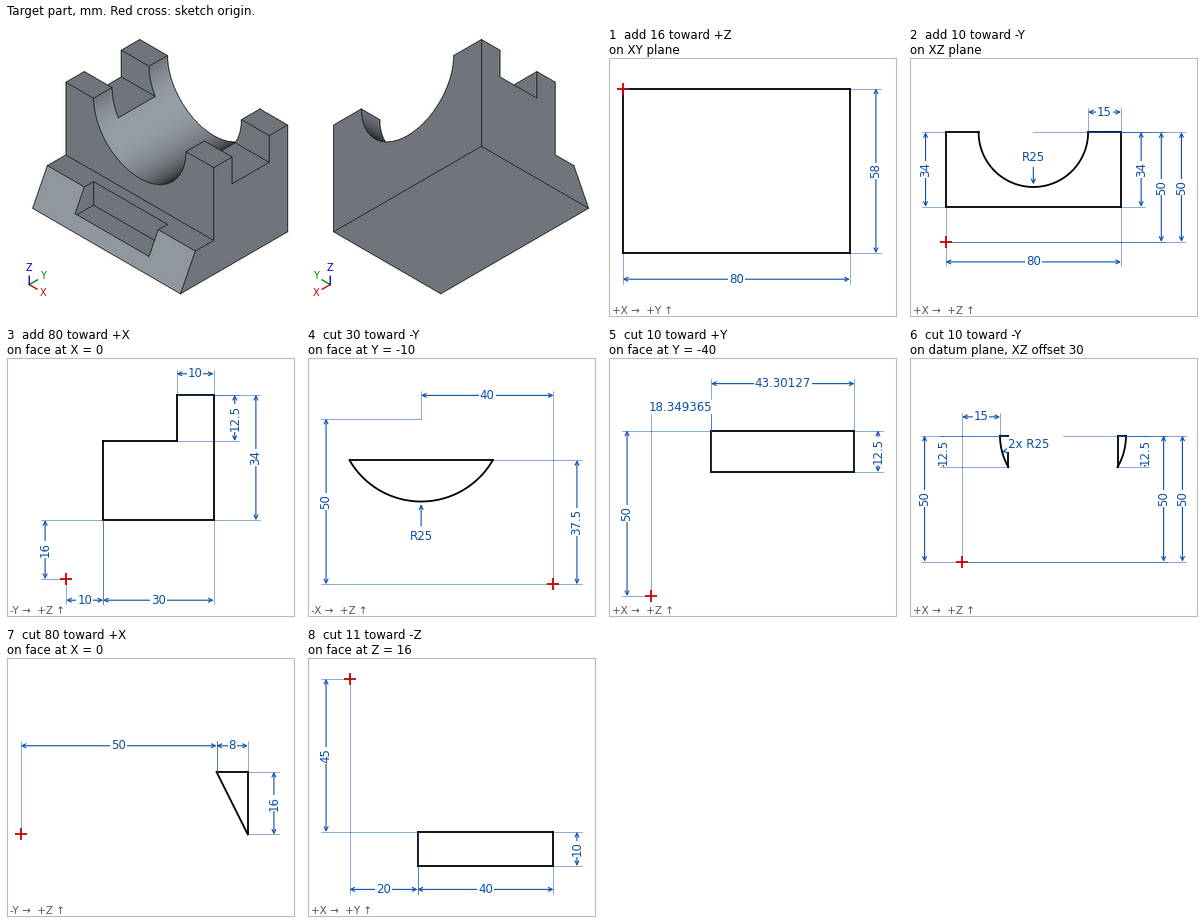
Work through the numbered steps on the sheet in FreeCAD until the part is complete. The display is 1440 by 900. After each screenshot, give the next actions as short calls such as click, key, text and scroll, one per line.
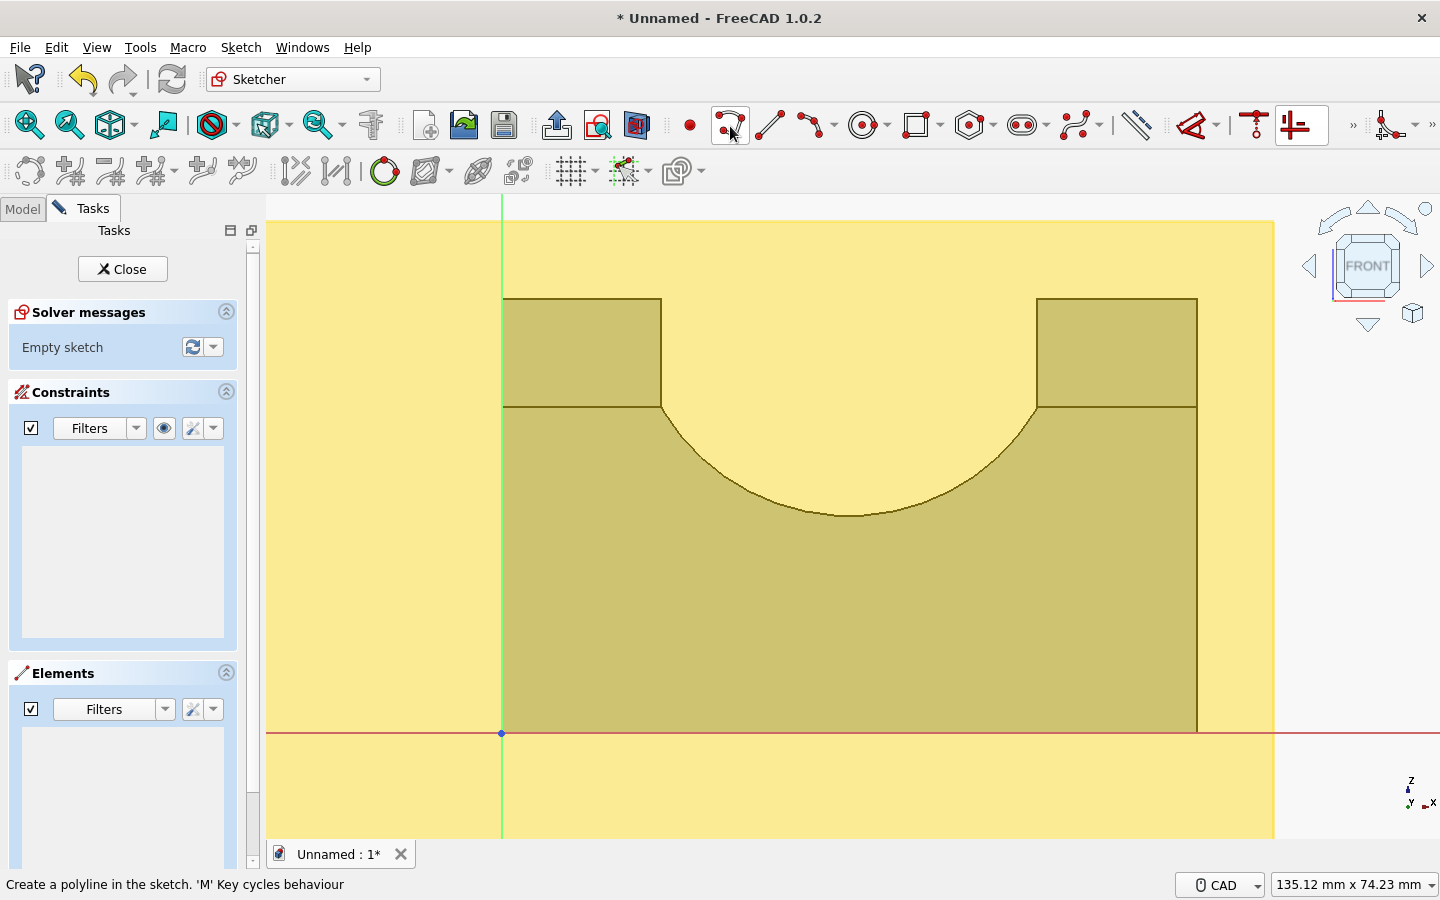
click(632, 299)
click(661, 299)
click(661, 407)
right_click(661, 407)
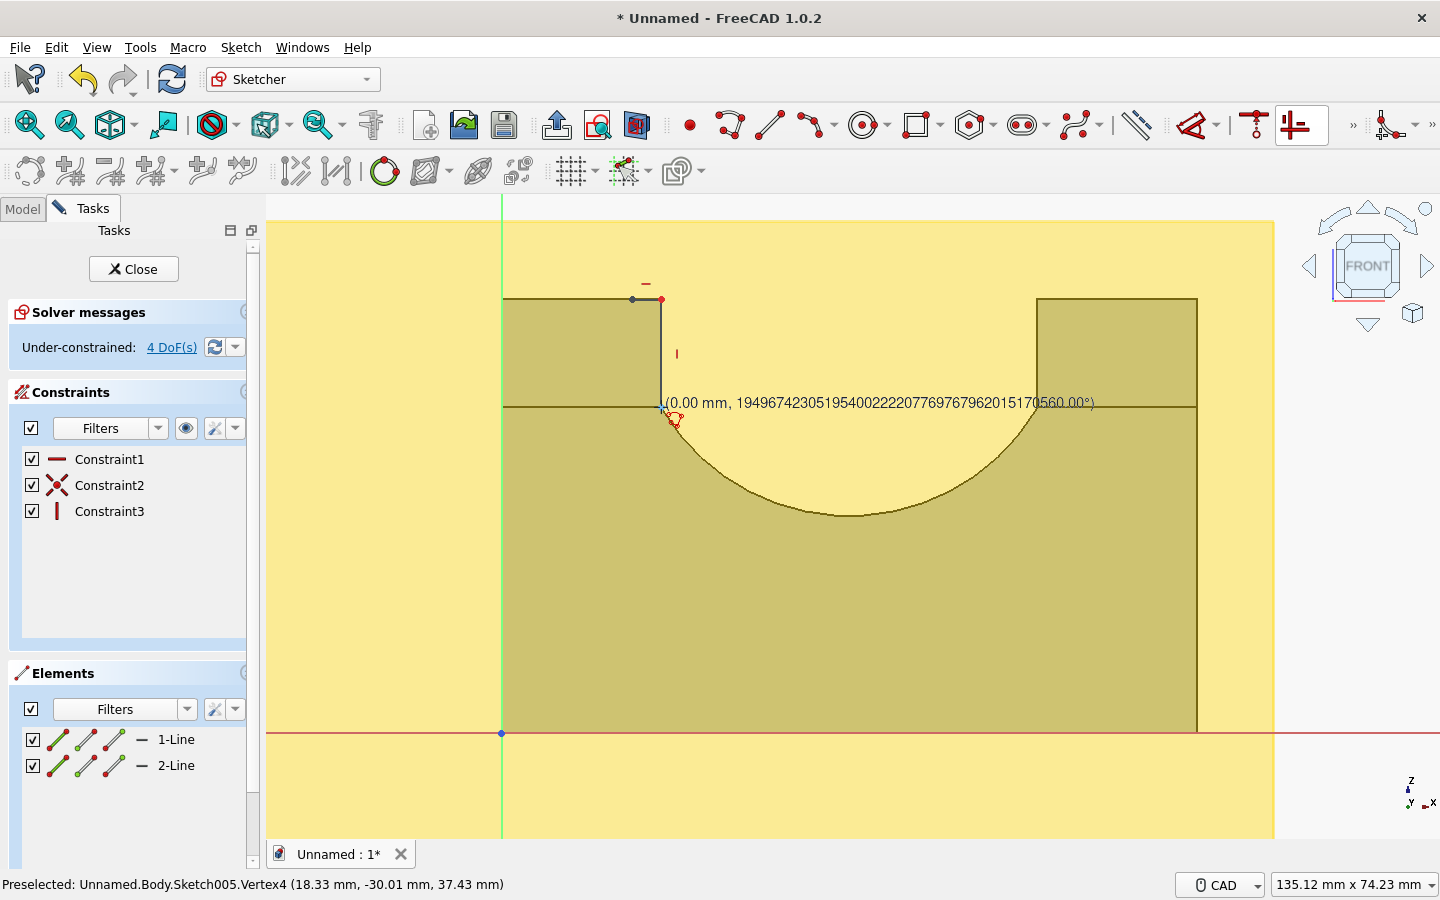
click(810, 126)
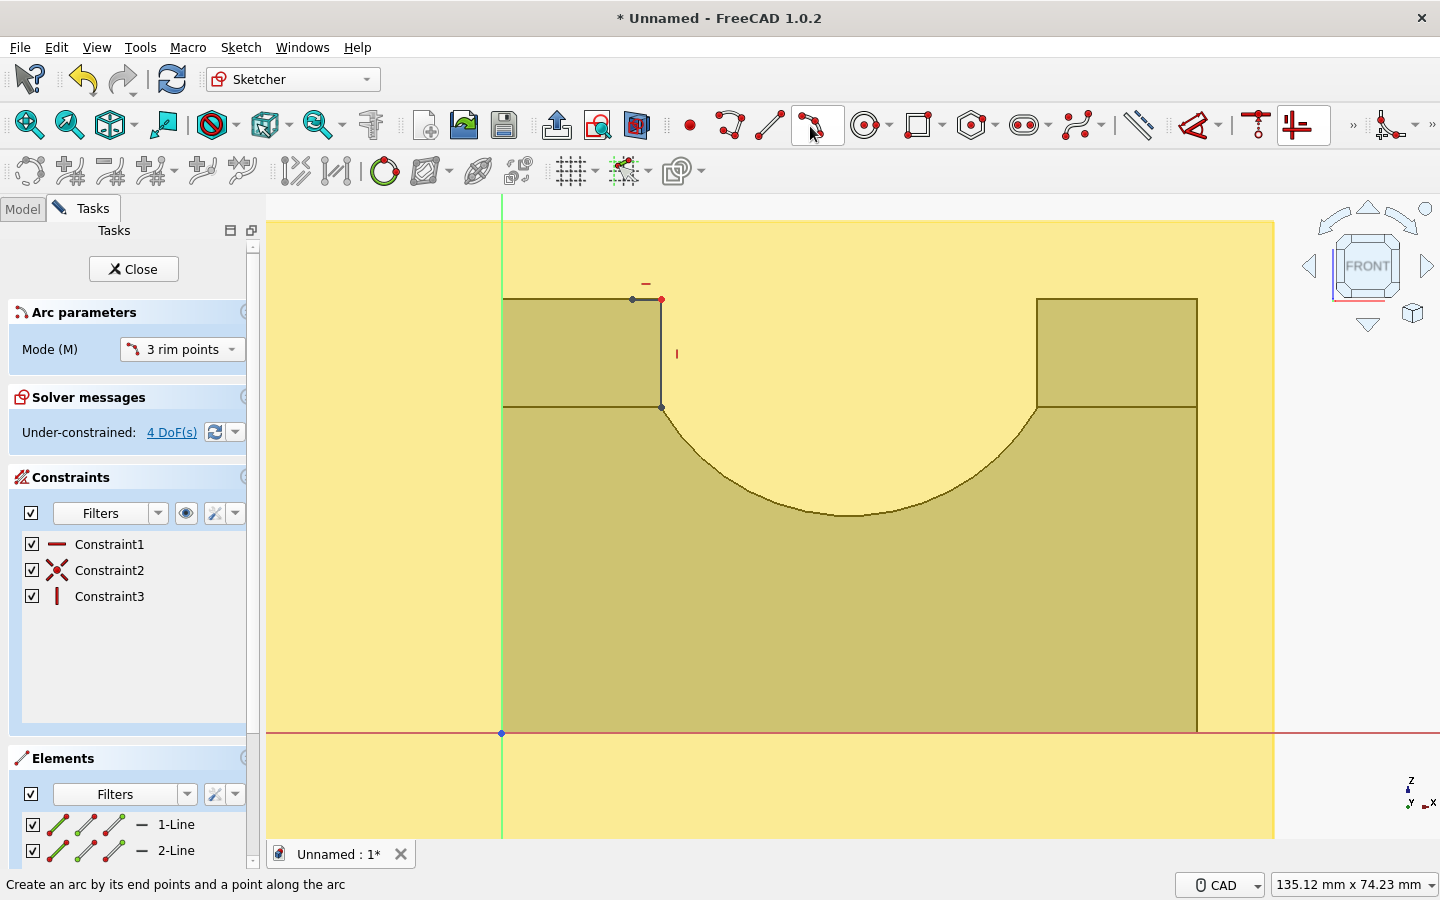
click(661, 408)
click(632, 300)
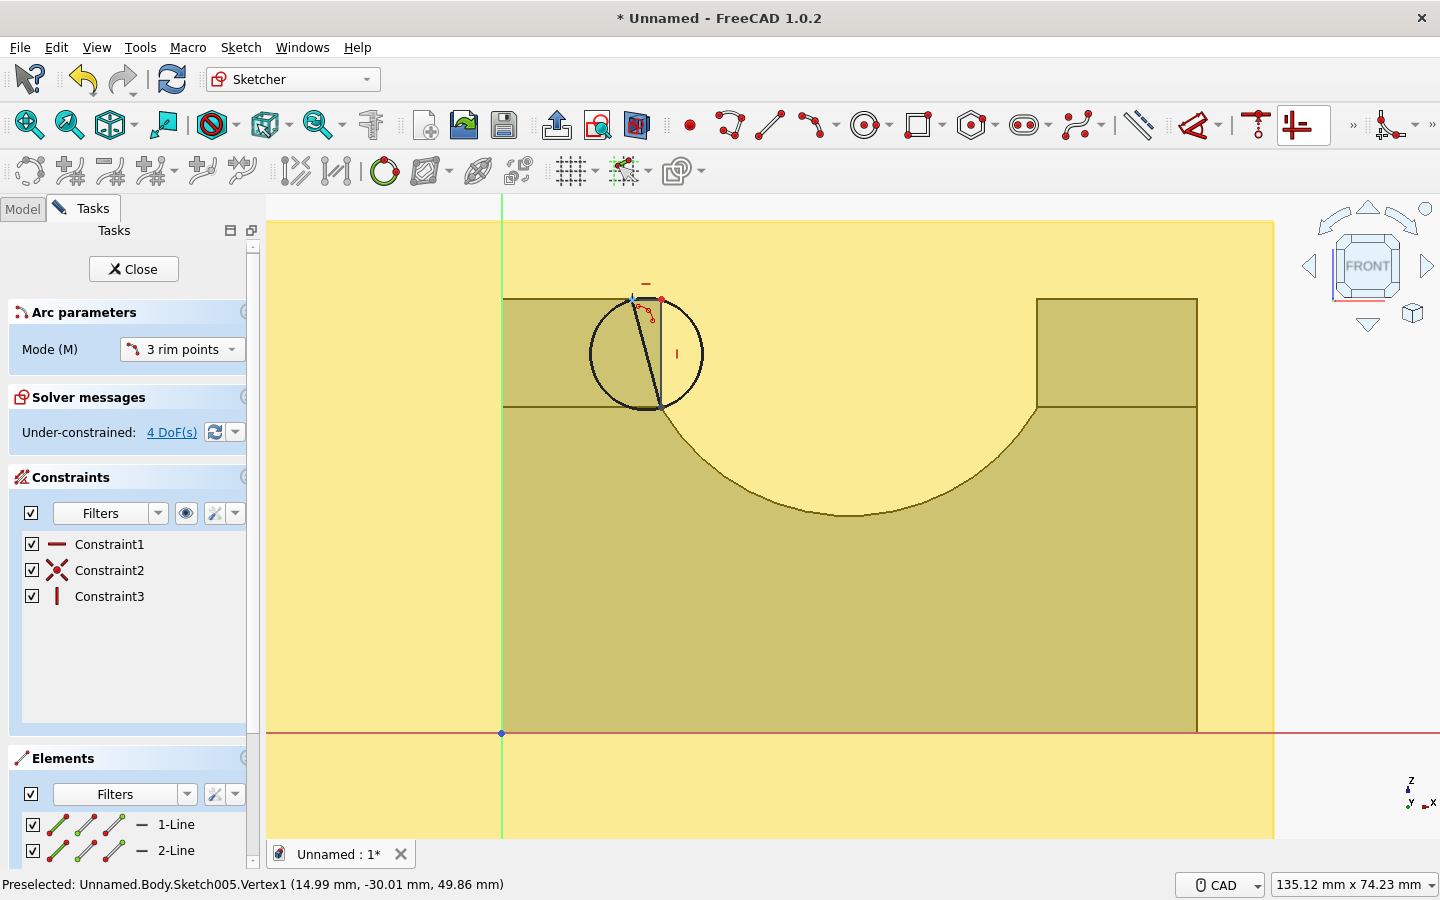
scroll(639, 355, up, 4)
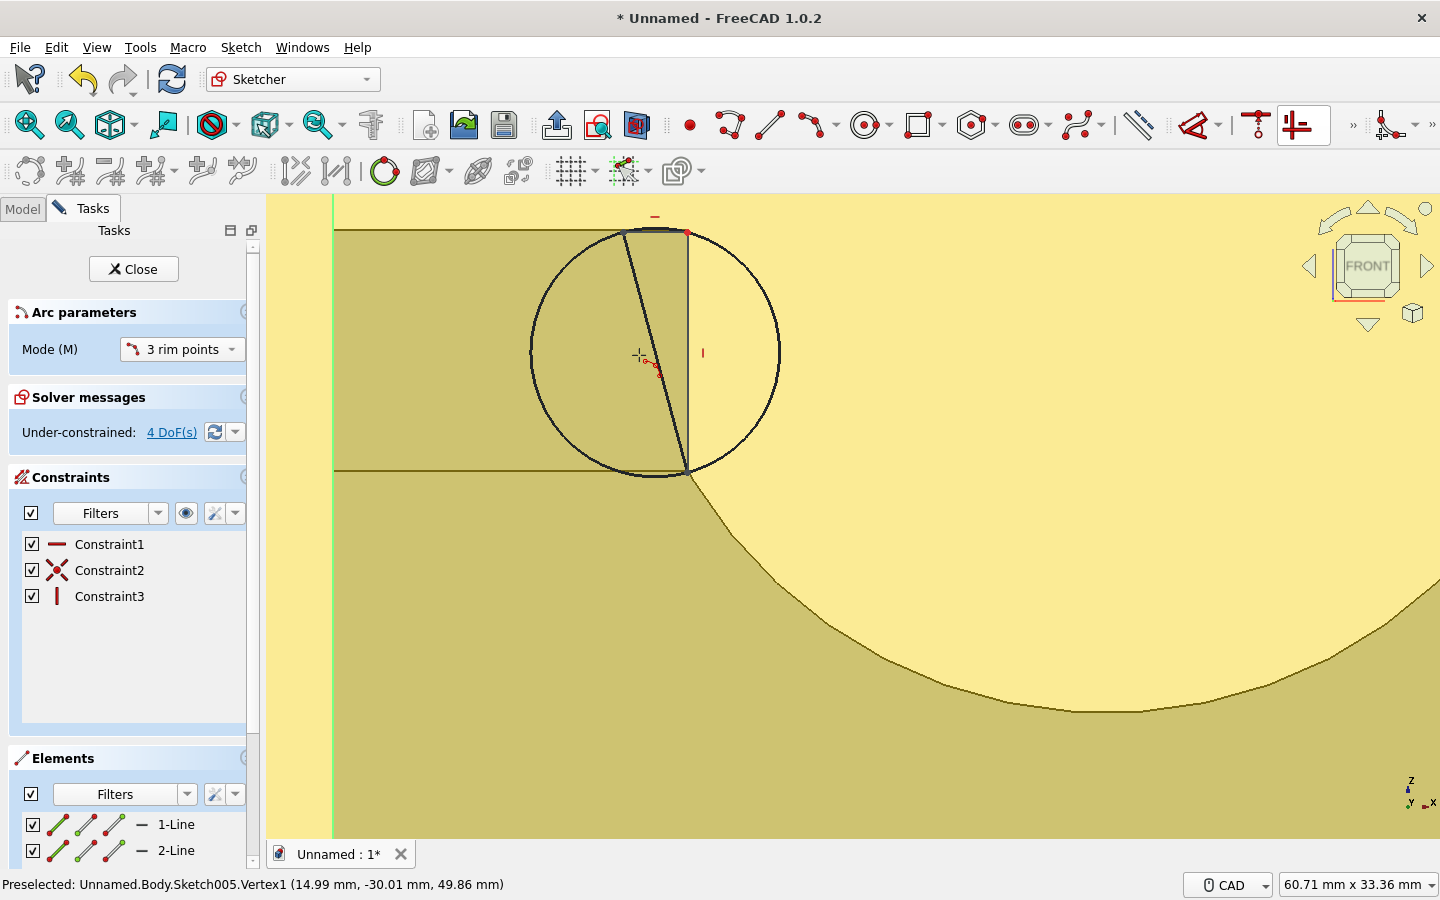
click(640, 355)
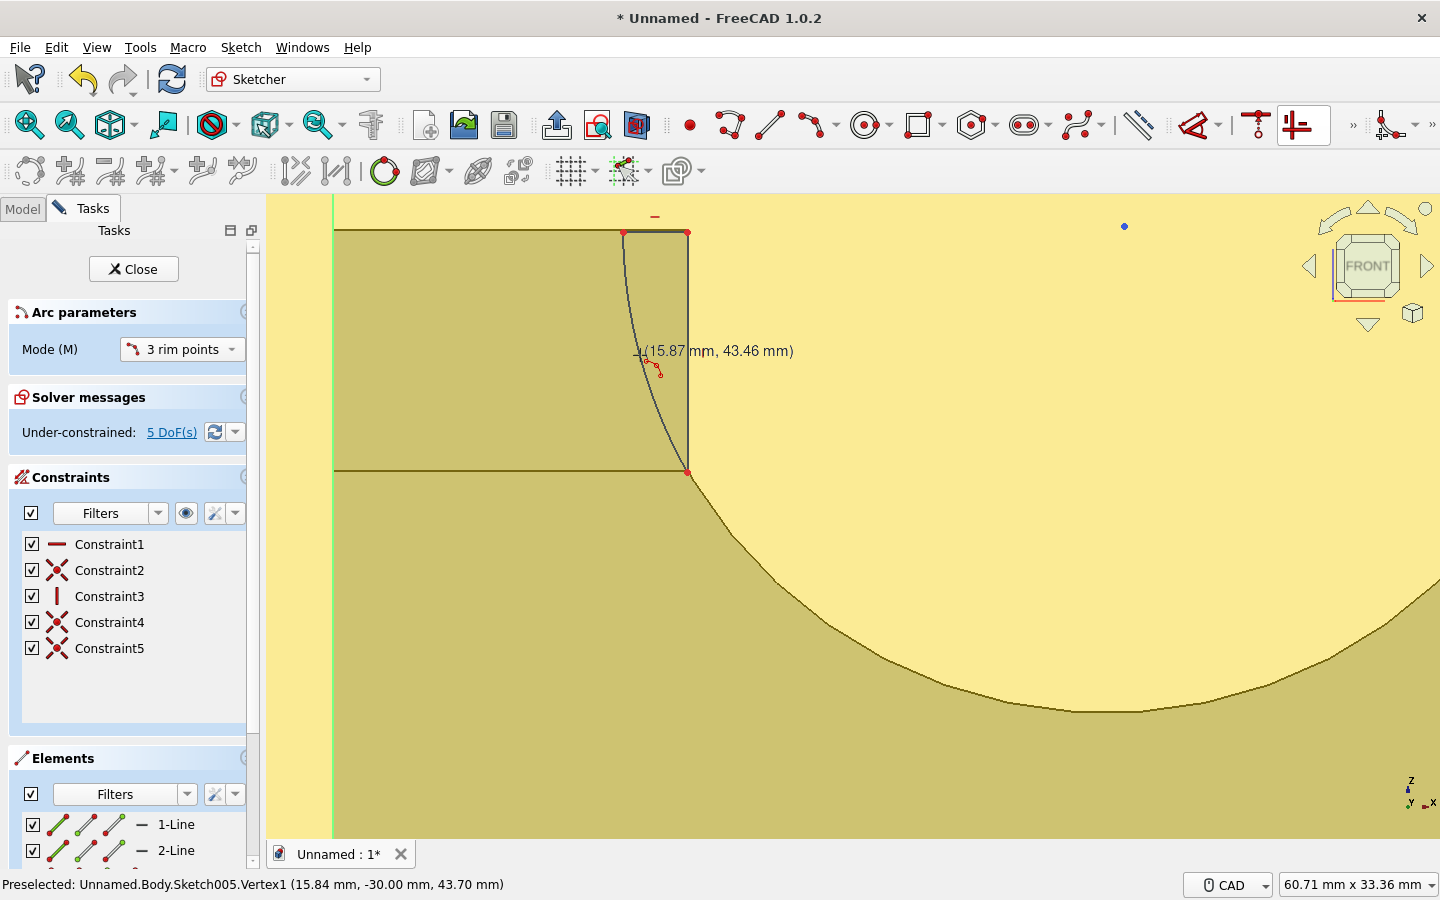
click(730, 126)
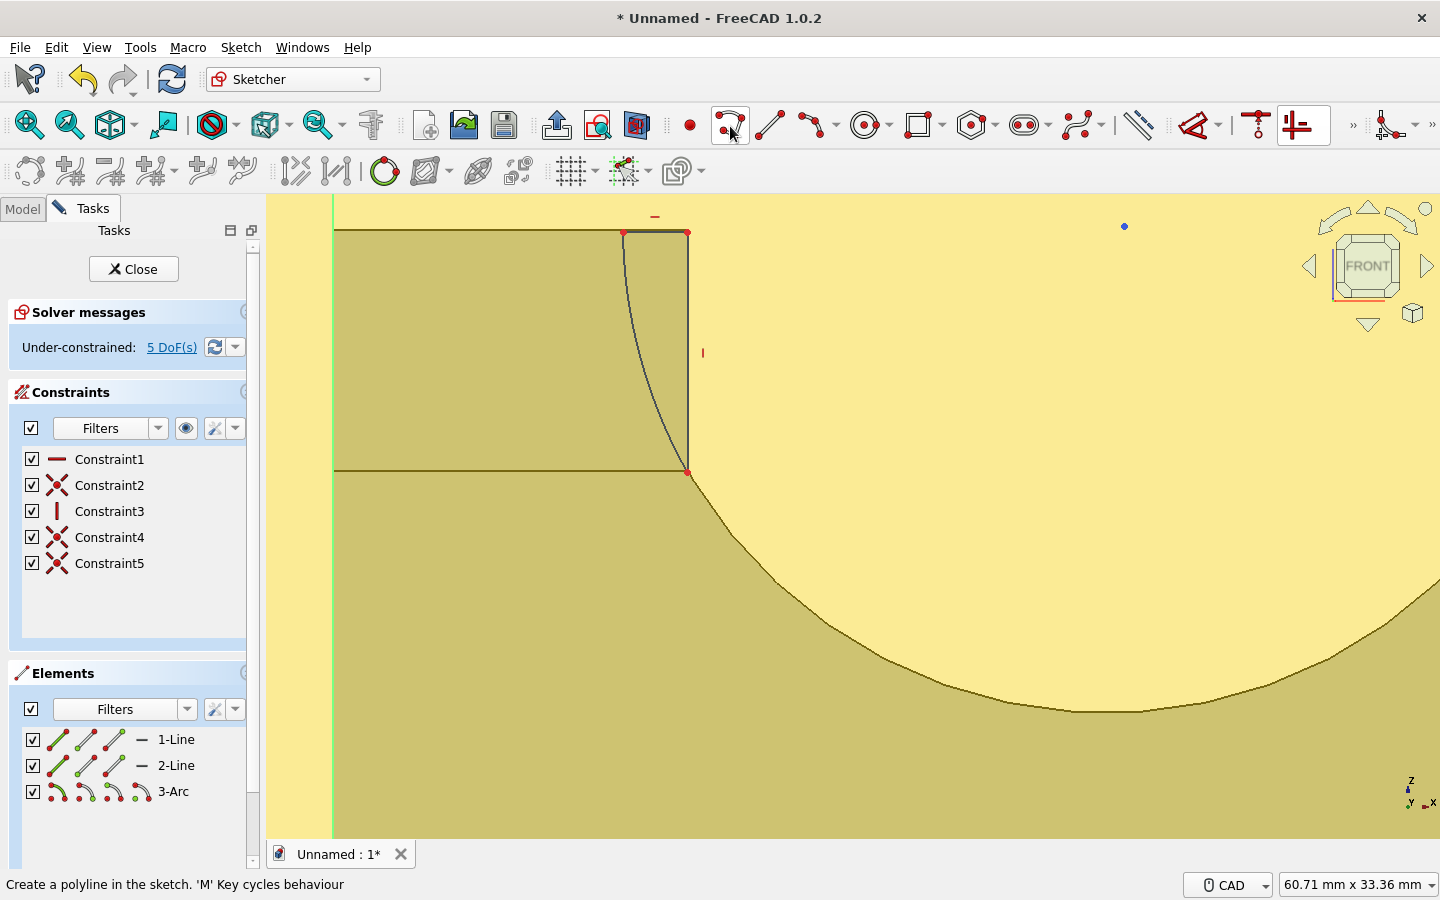
scroll(640, 356, down, 4)